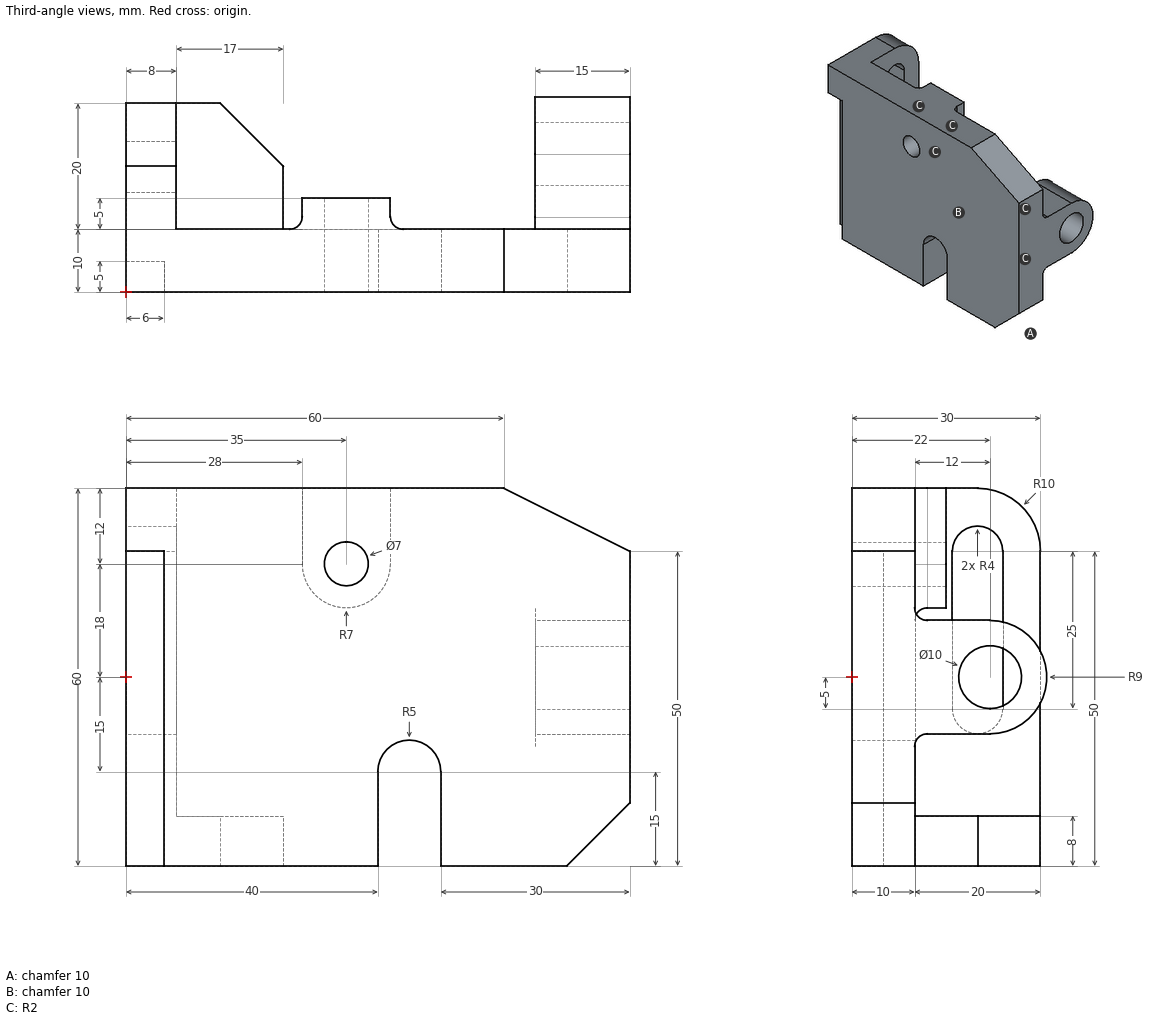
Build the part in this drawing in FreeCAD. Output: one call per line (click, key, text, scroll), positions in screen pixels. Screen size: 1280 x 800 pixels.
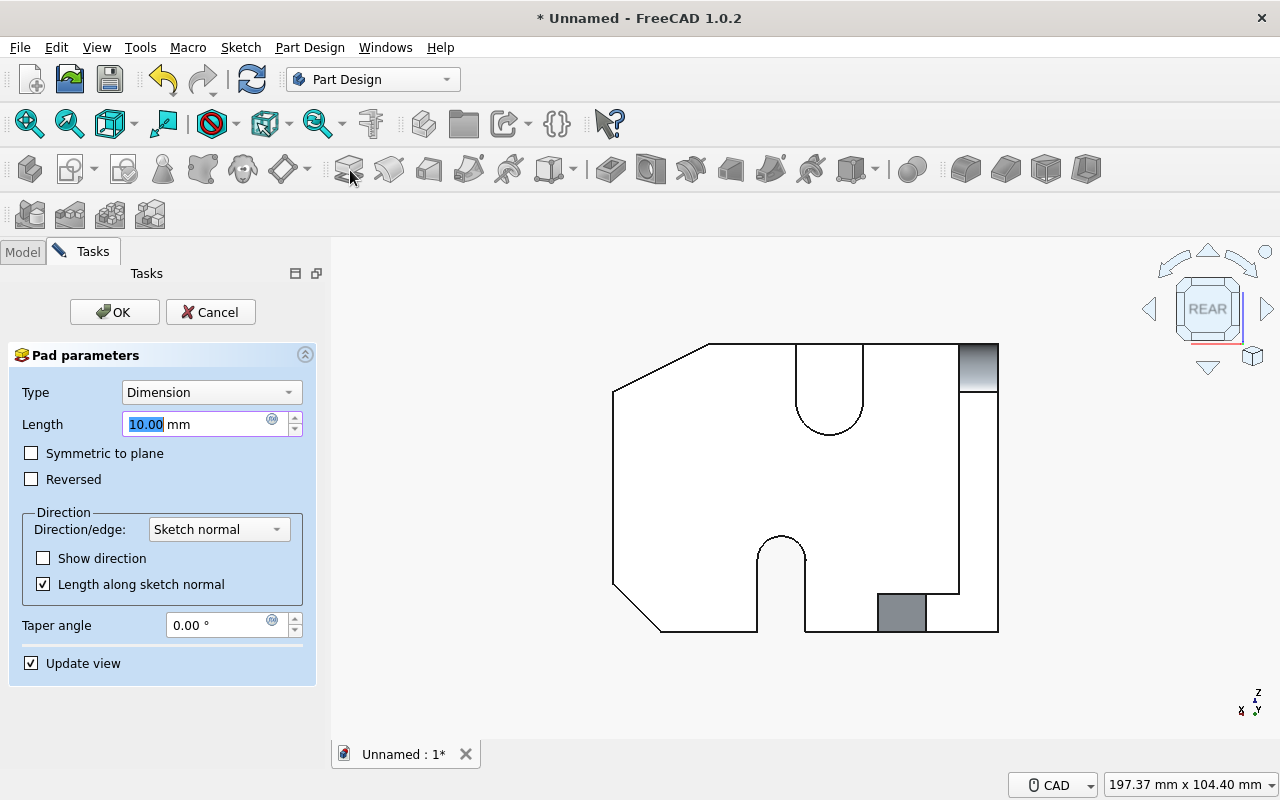
text(5)
key(Tab)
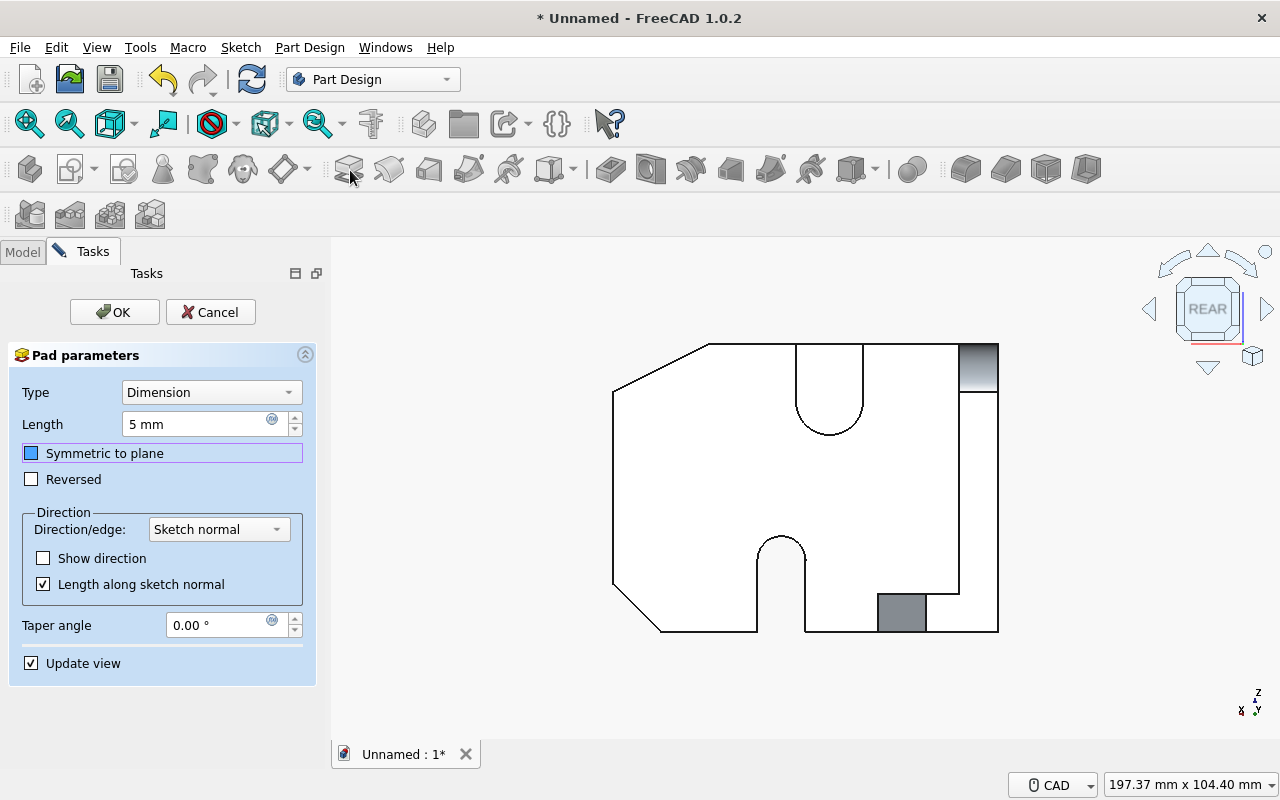
click(115, 312)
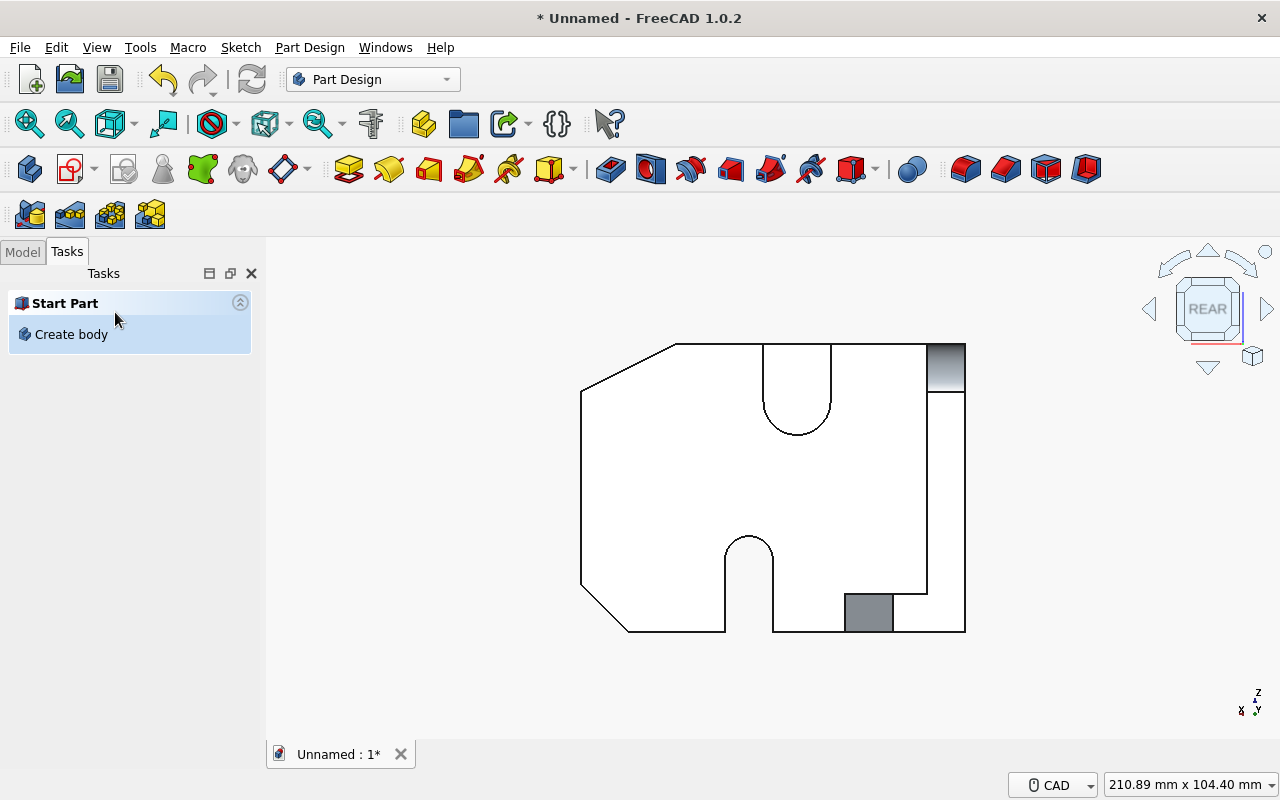
click(797, 388)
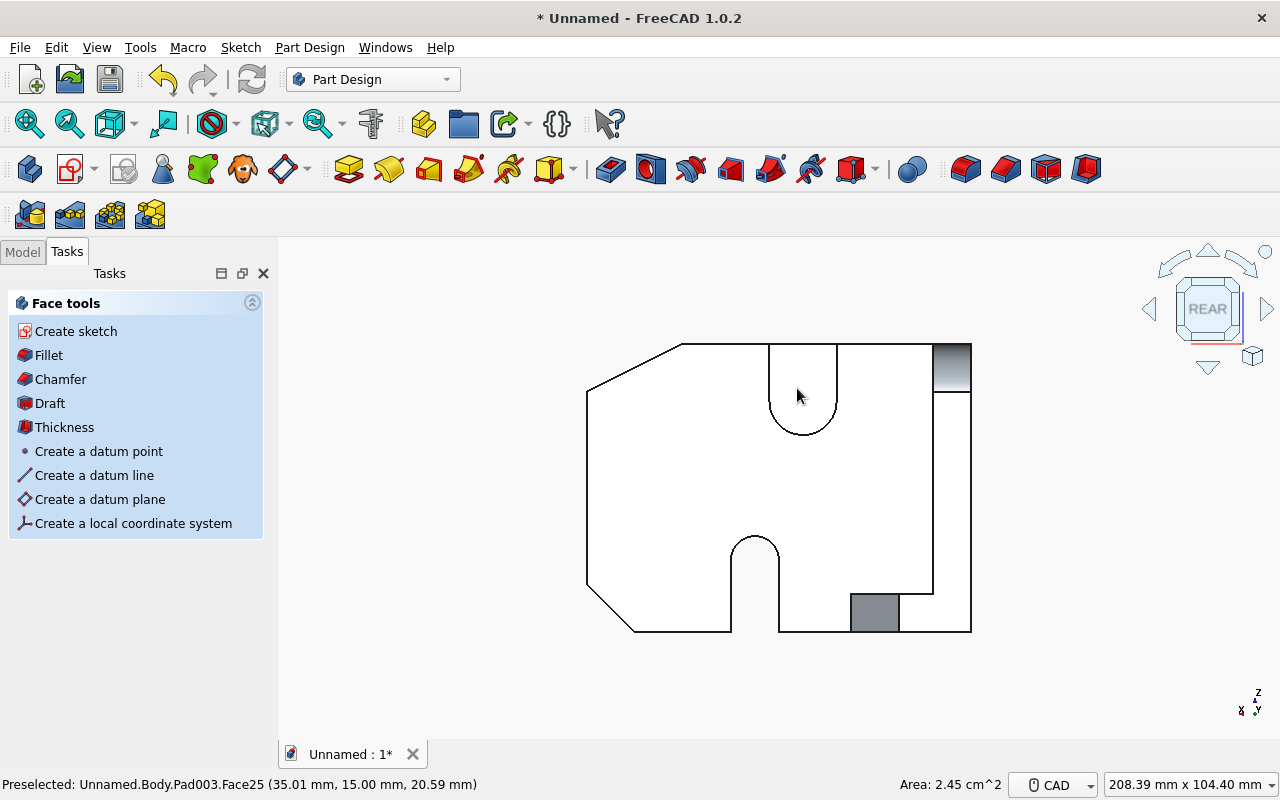
click(70, 170)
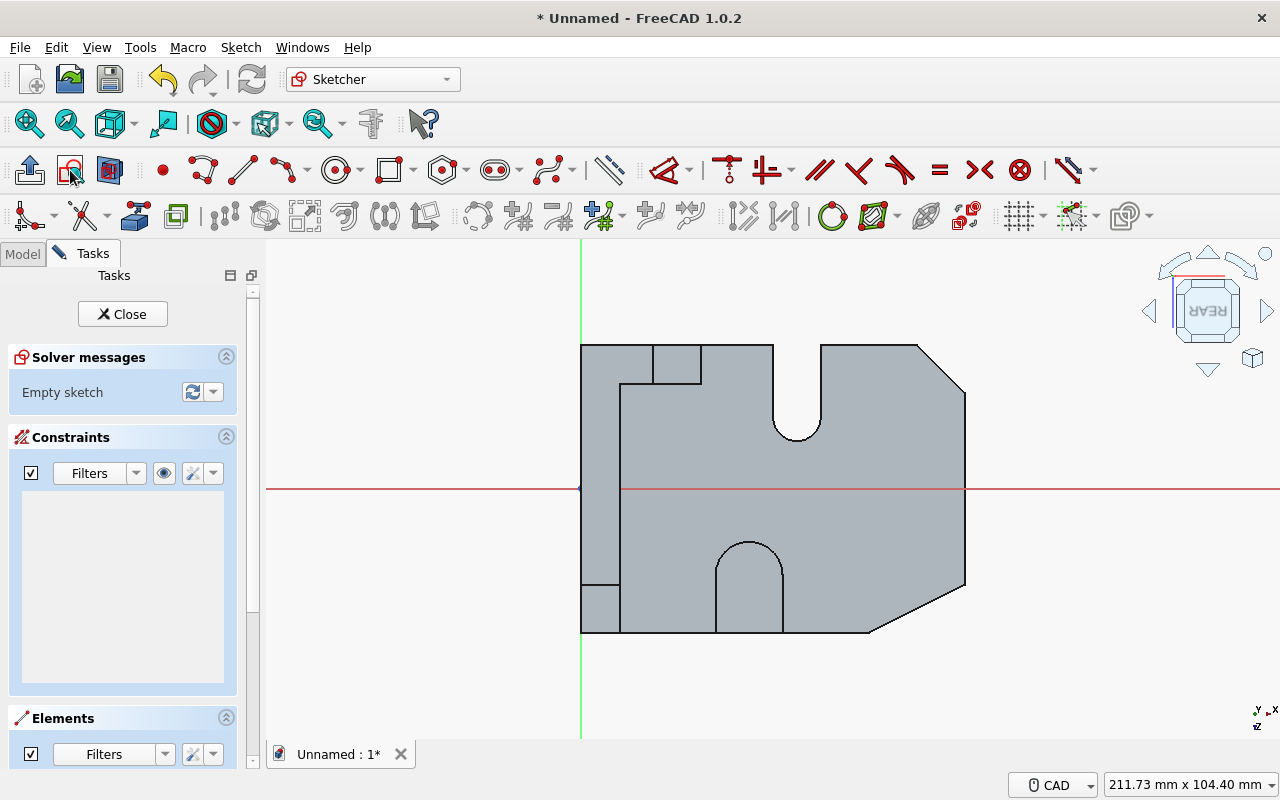
scroll(755, 586, up, 11)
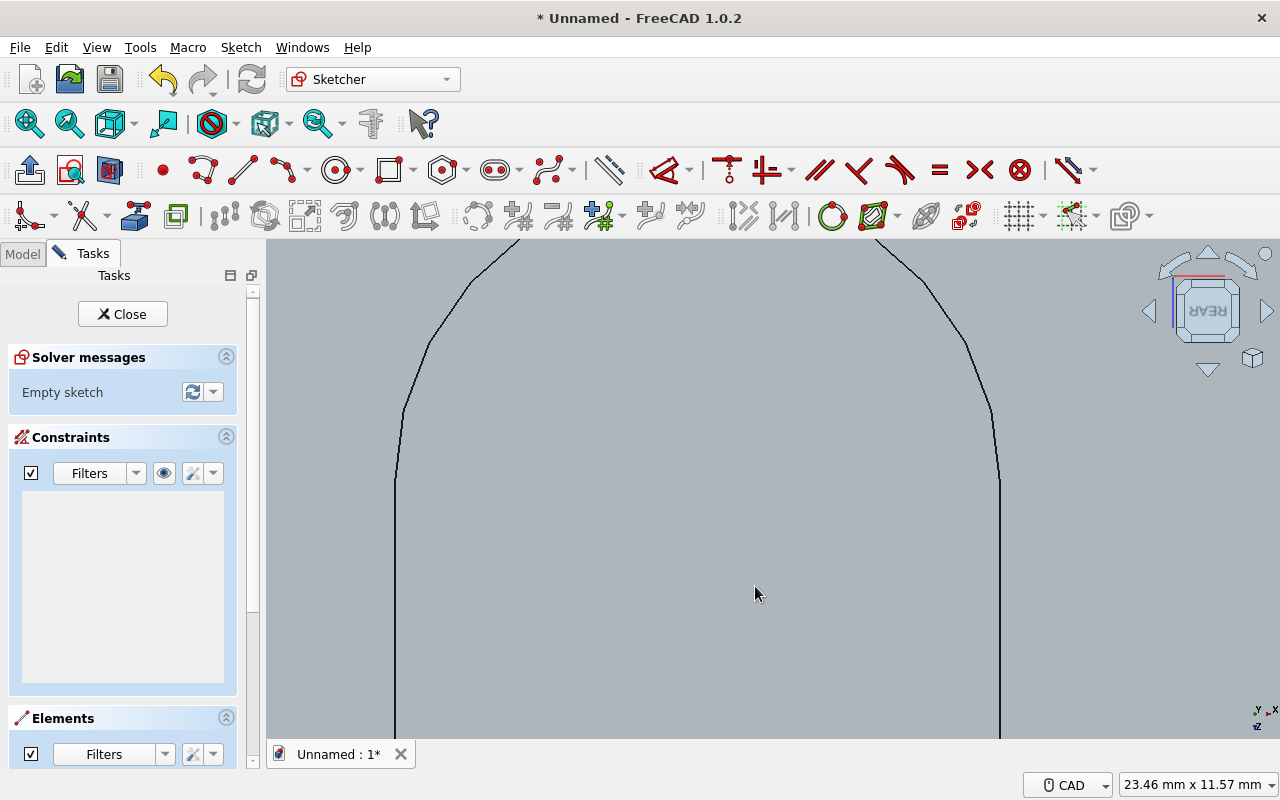
click(336, 170)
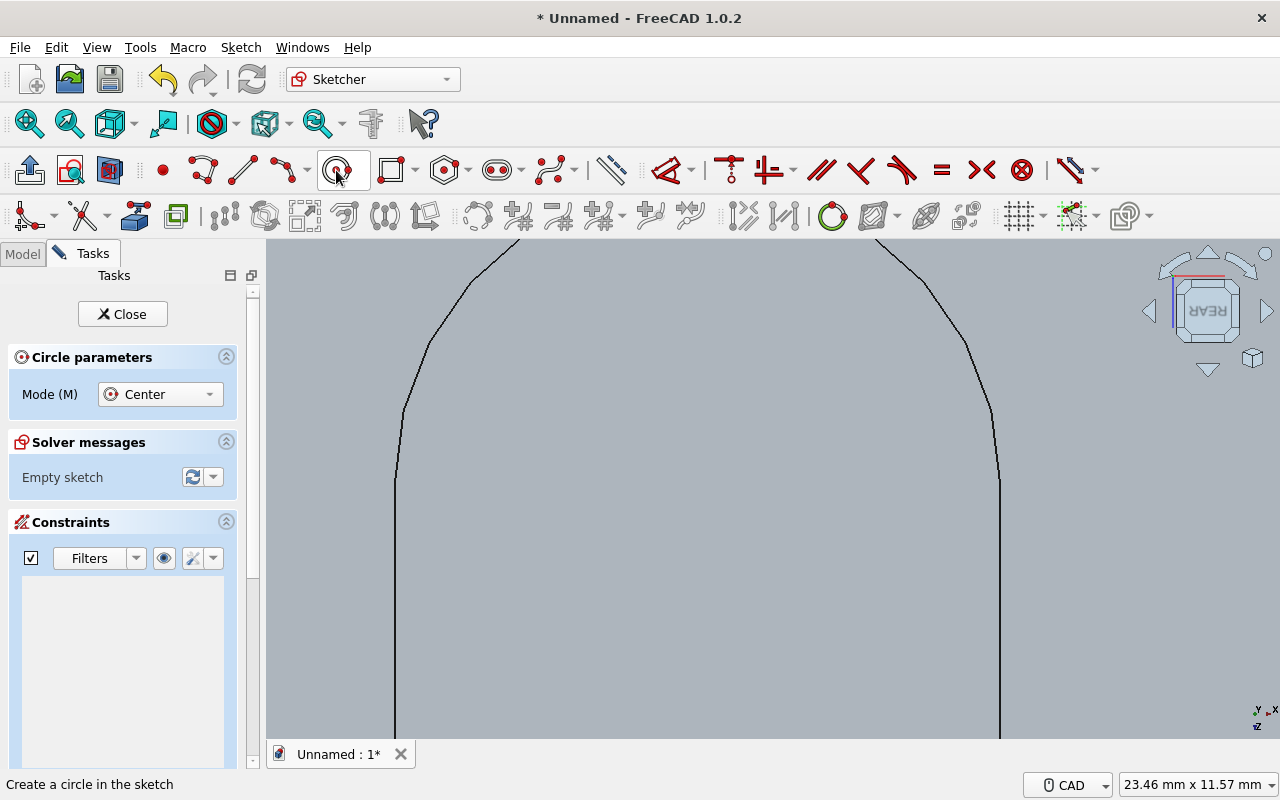
click(697, 483)
click(804, 376)
key(Escape)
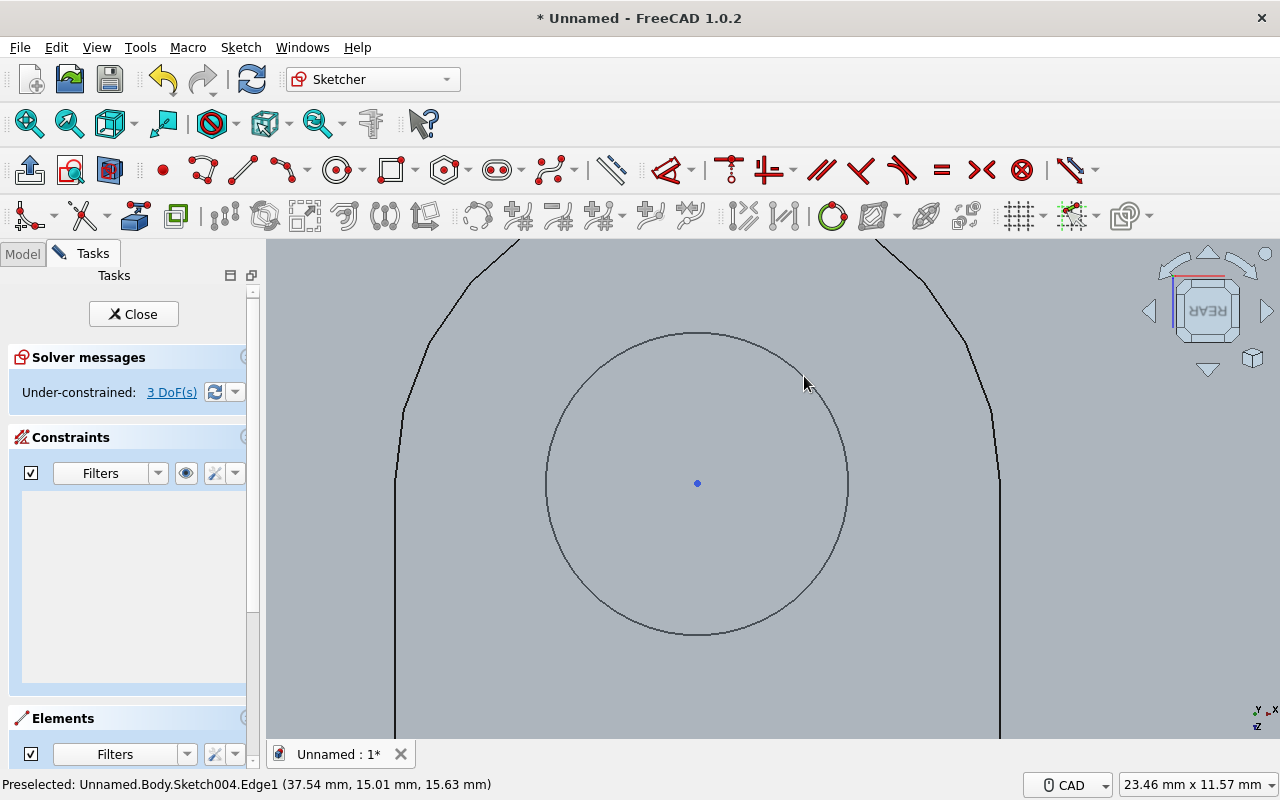
click(666, 170)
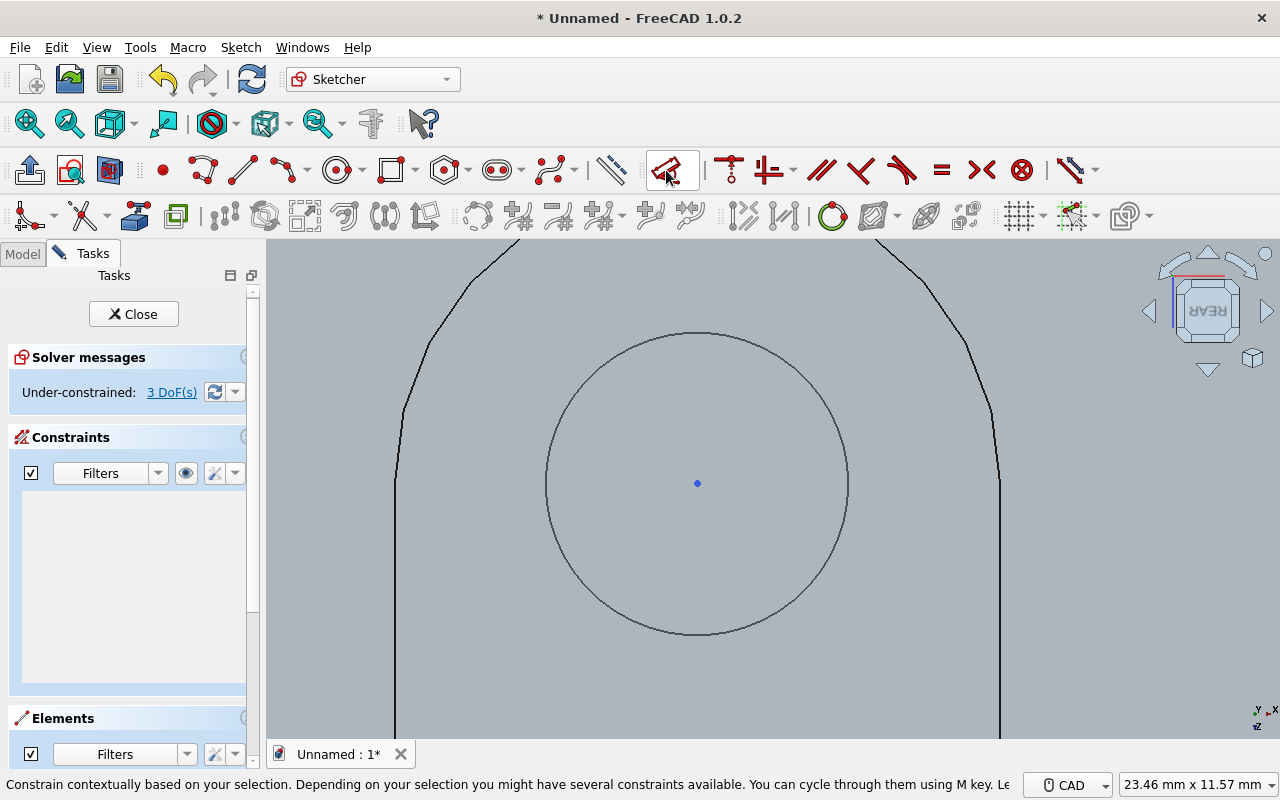
click(804, 377)
click(827, 354)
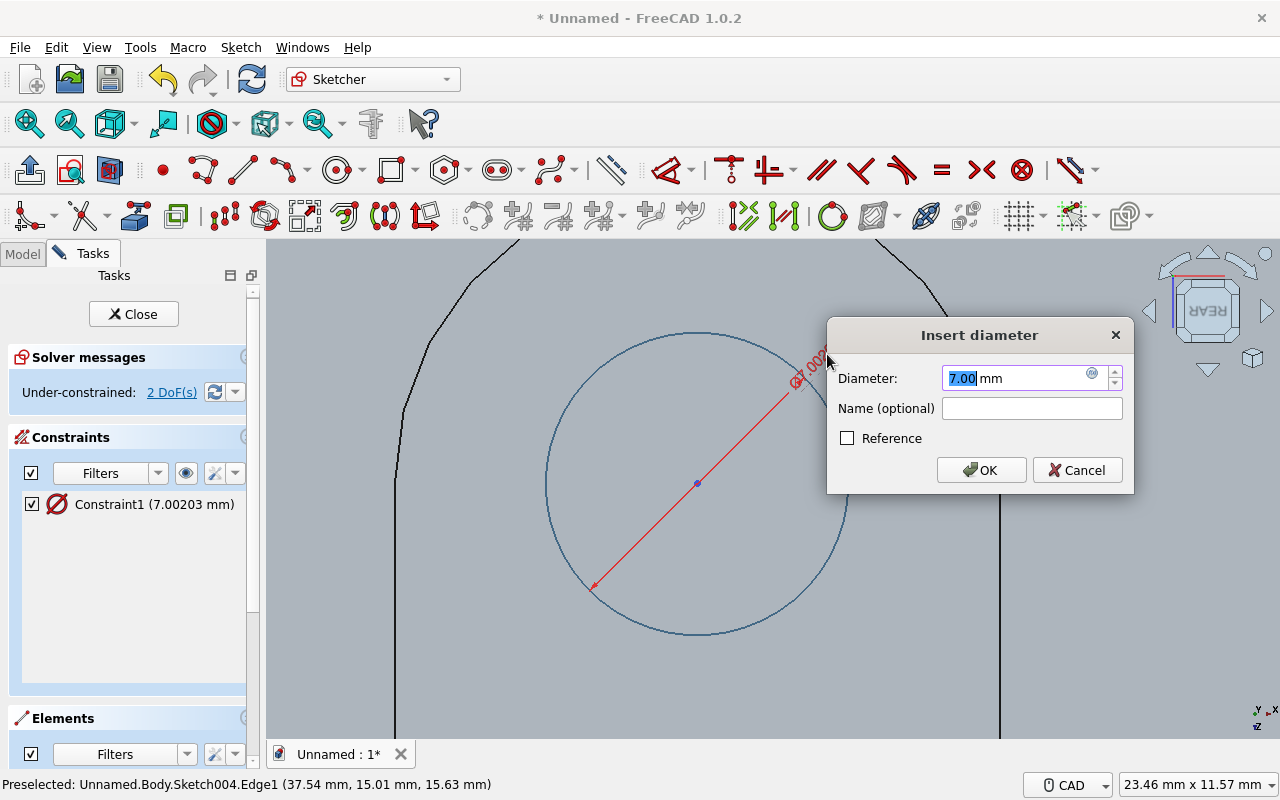
text(7)
key(Return)